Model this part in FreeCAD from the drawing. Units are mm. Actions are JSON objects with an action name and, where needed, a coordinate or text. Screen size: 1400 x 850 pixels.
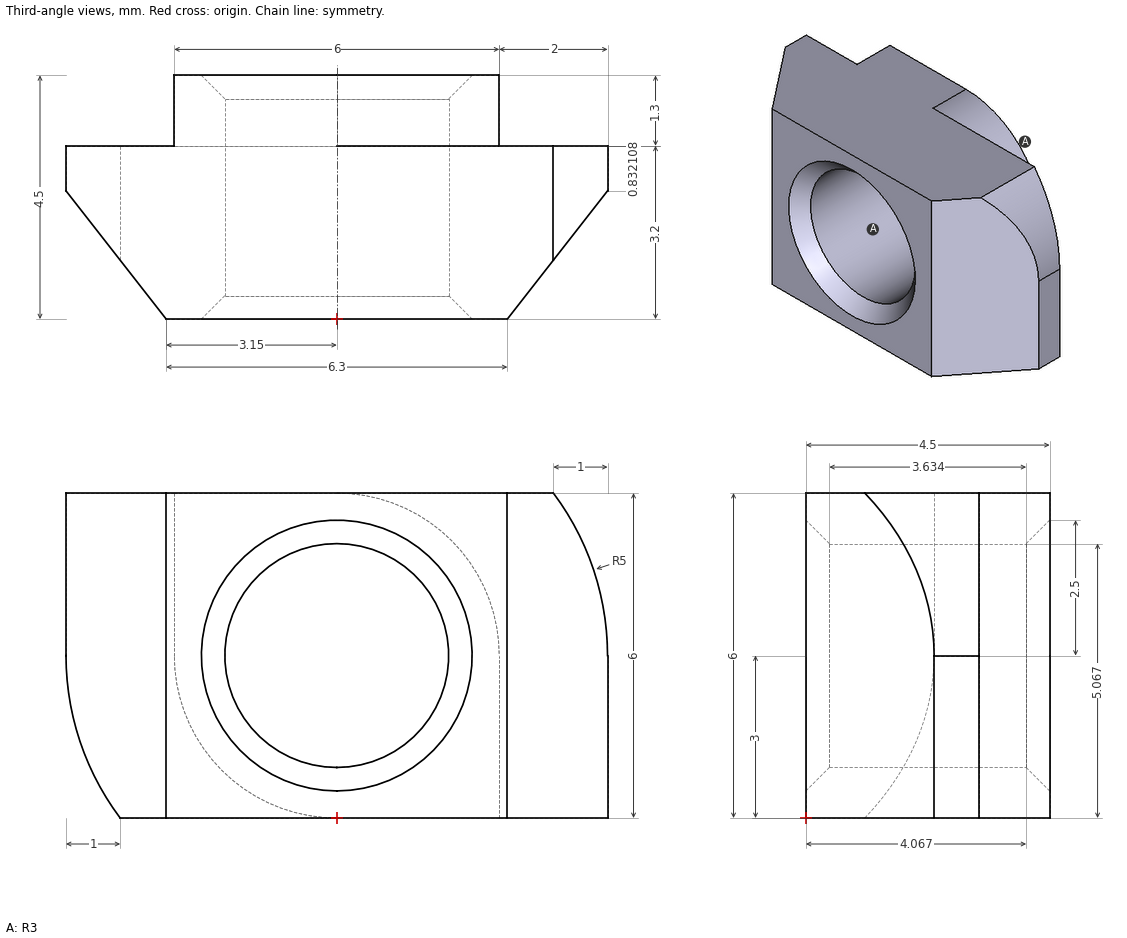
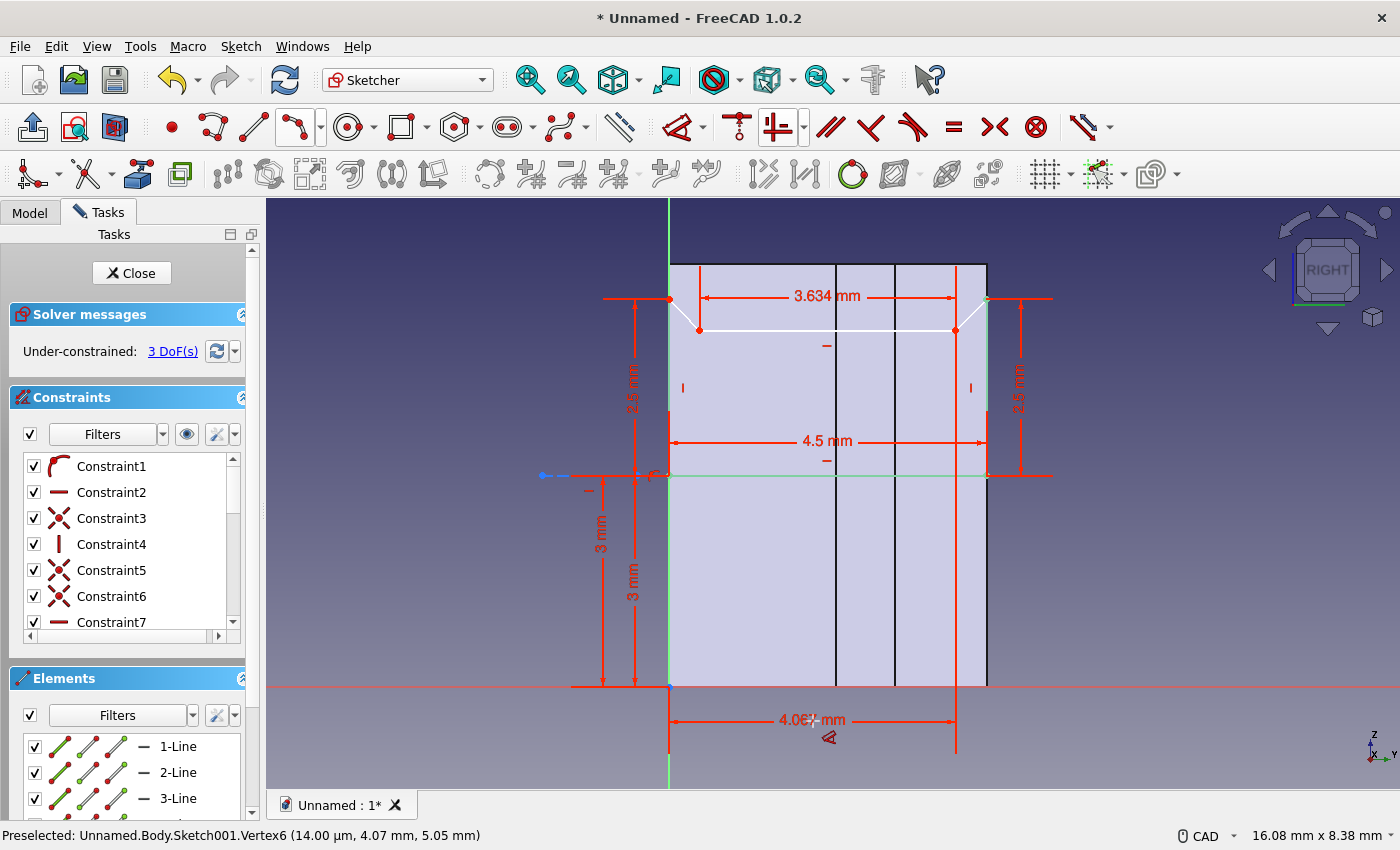
{"action": "left_click", "coordinate": [956, 331]}
{"action": "left_click", "coordinate": [990, 509]}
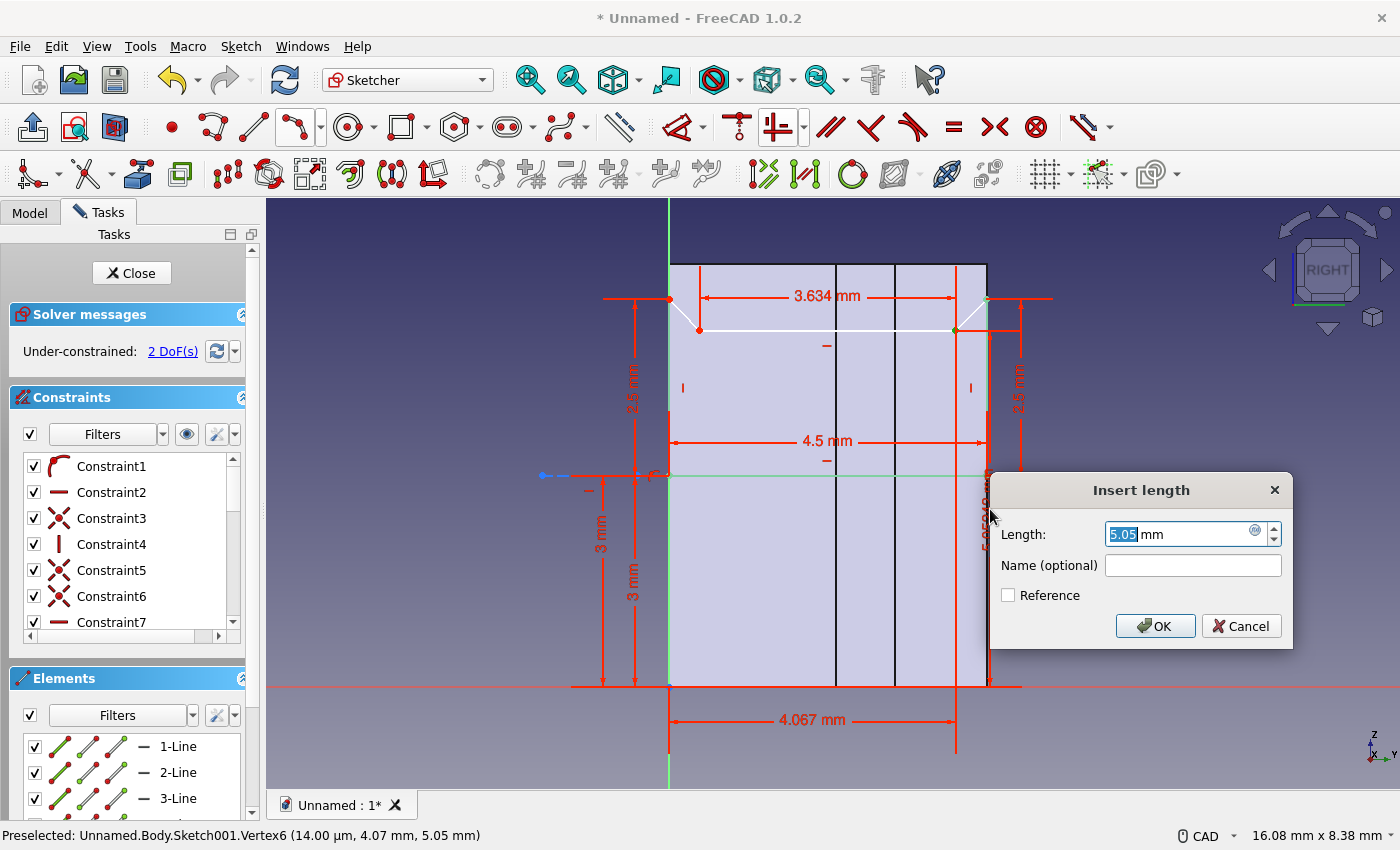
{"action": "type", "text": "5.067"}
{"action": "key", "text": "Return"}
{"action": "key", "text": "Escape"}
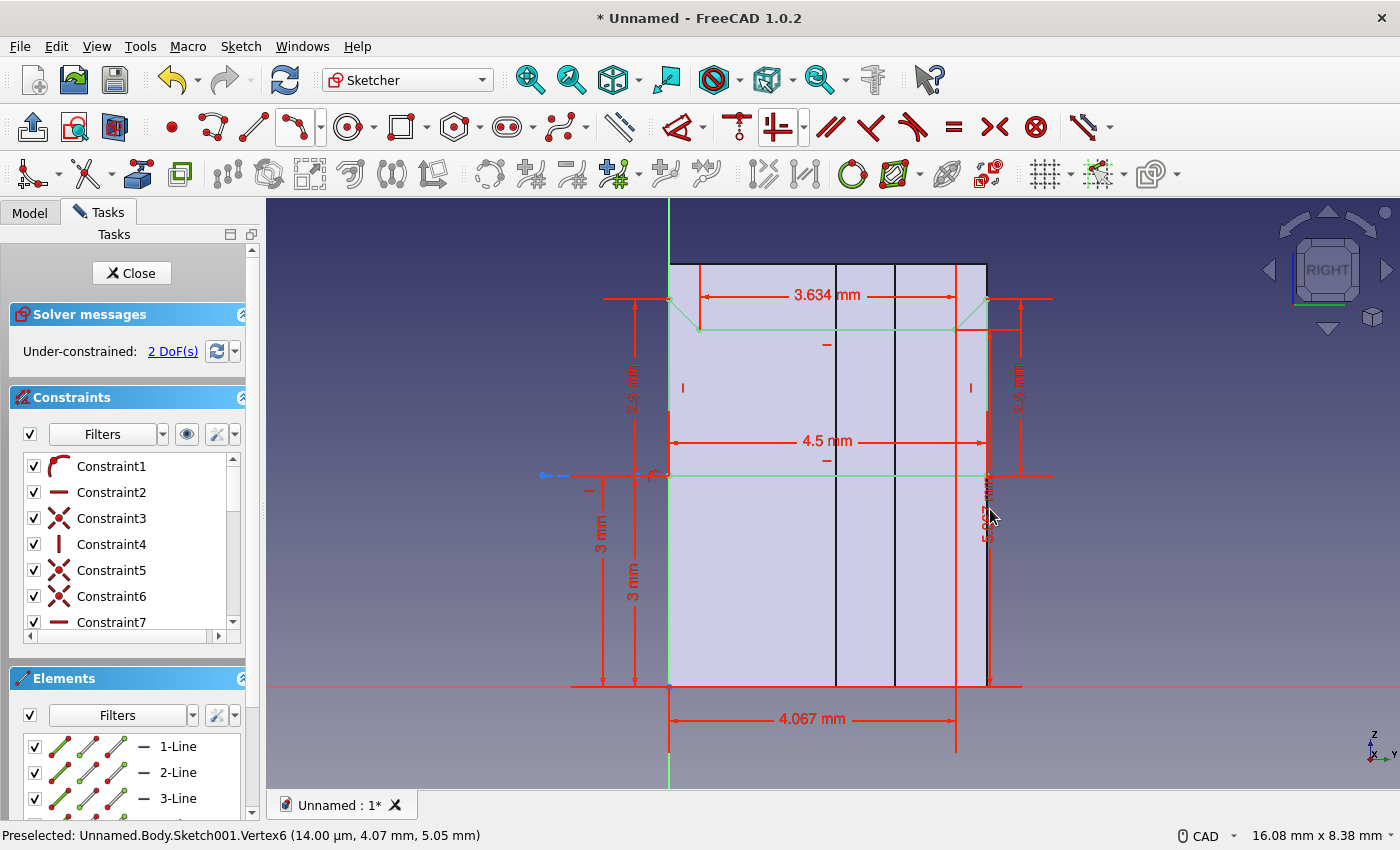
{"action": "left_click", "coordinate": [132, 273]}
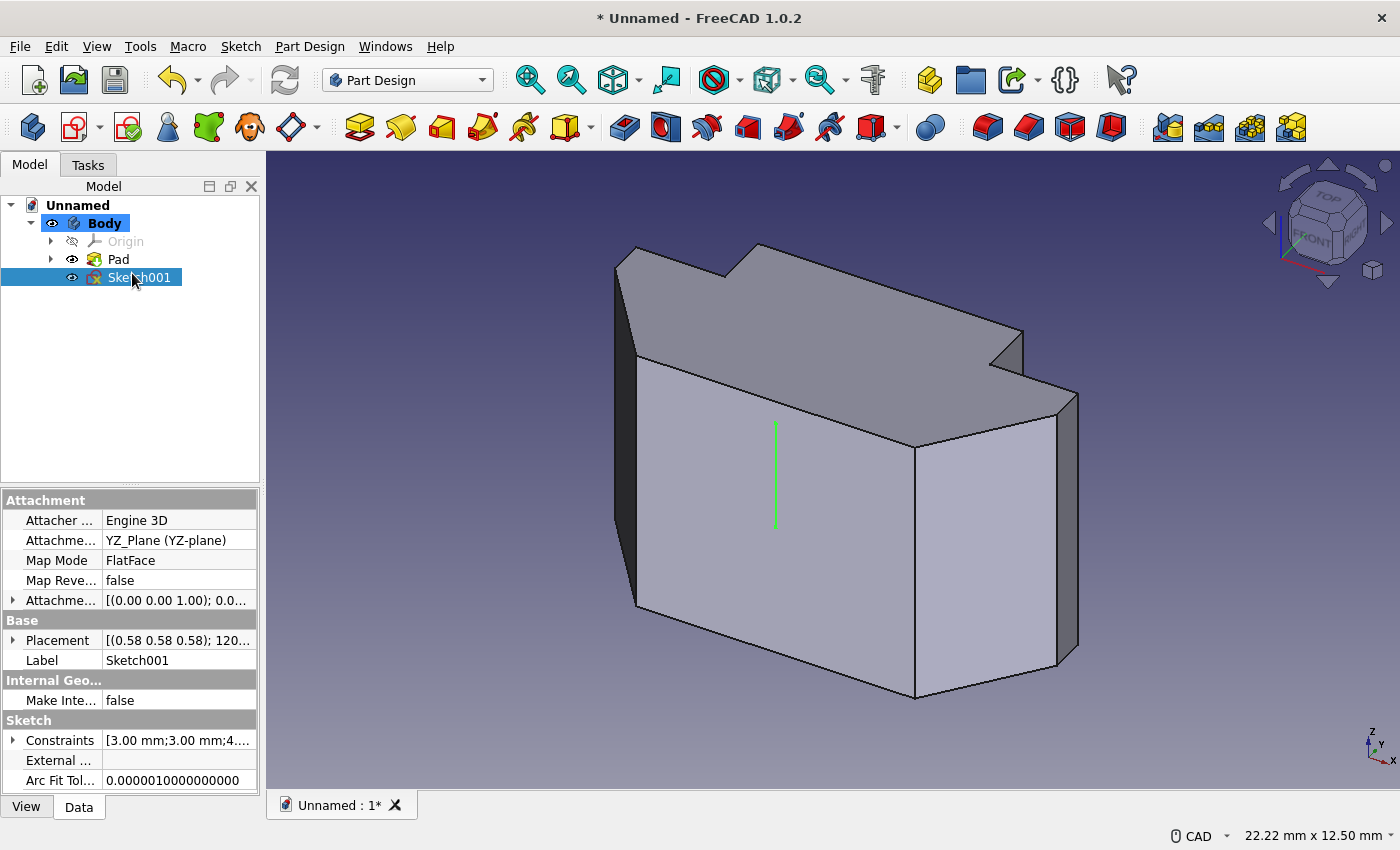
{"action": "left_click", "coordinate": [707, 128]}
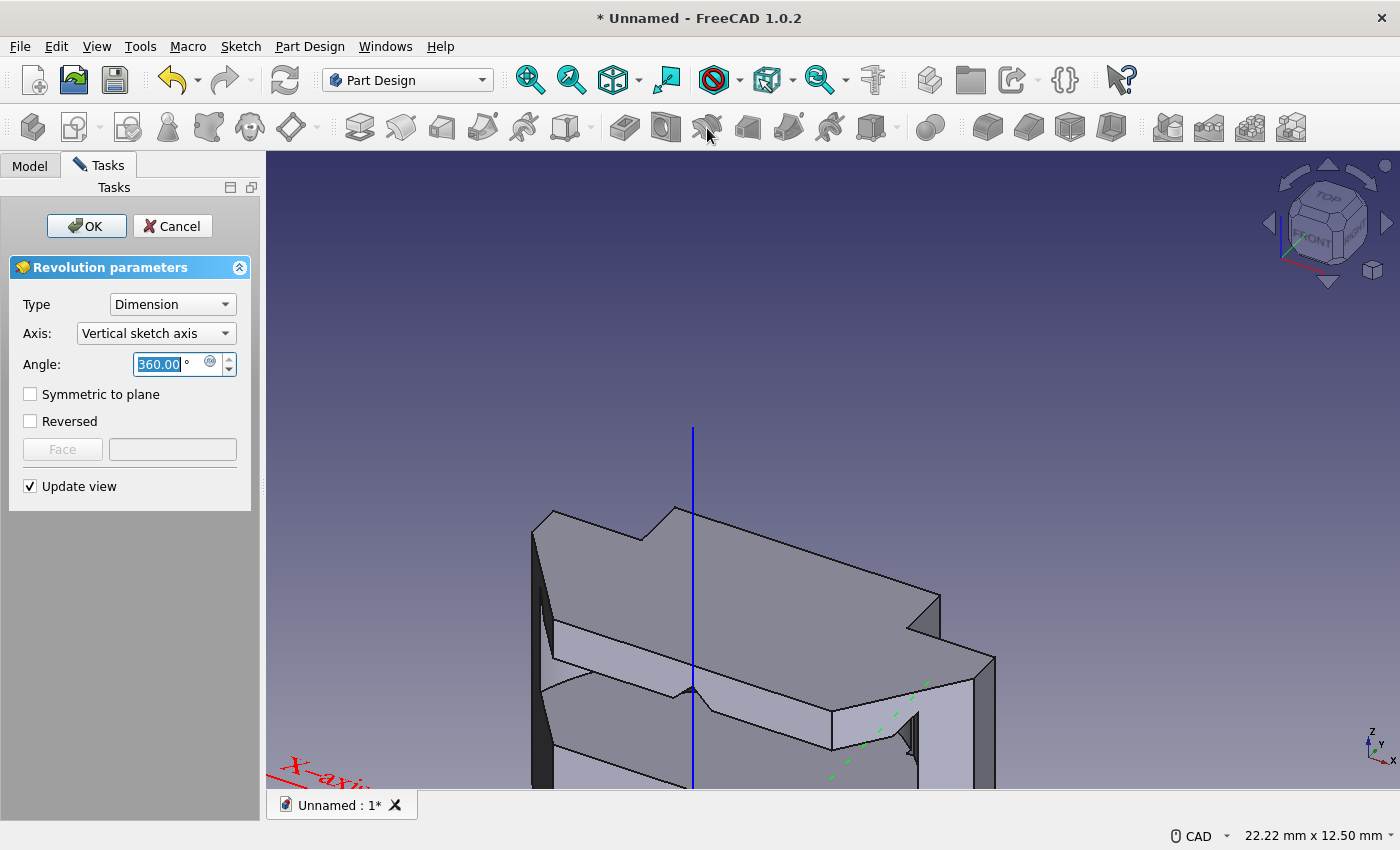
{"action": "left_click", "coordinate": [157, 334]}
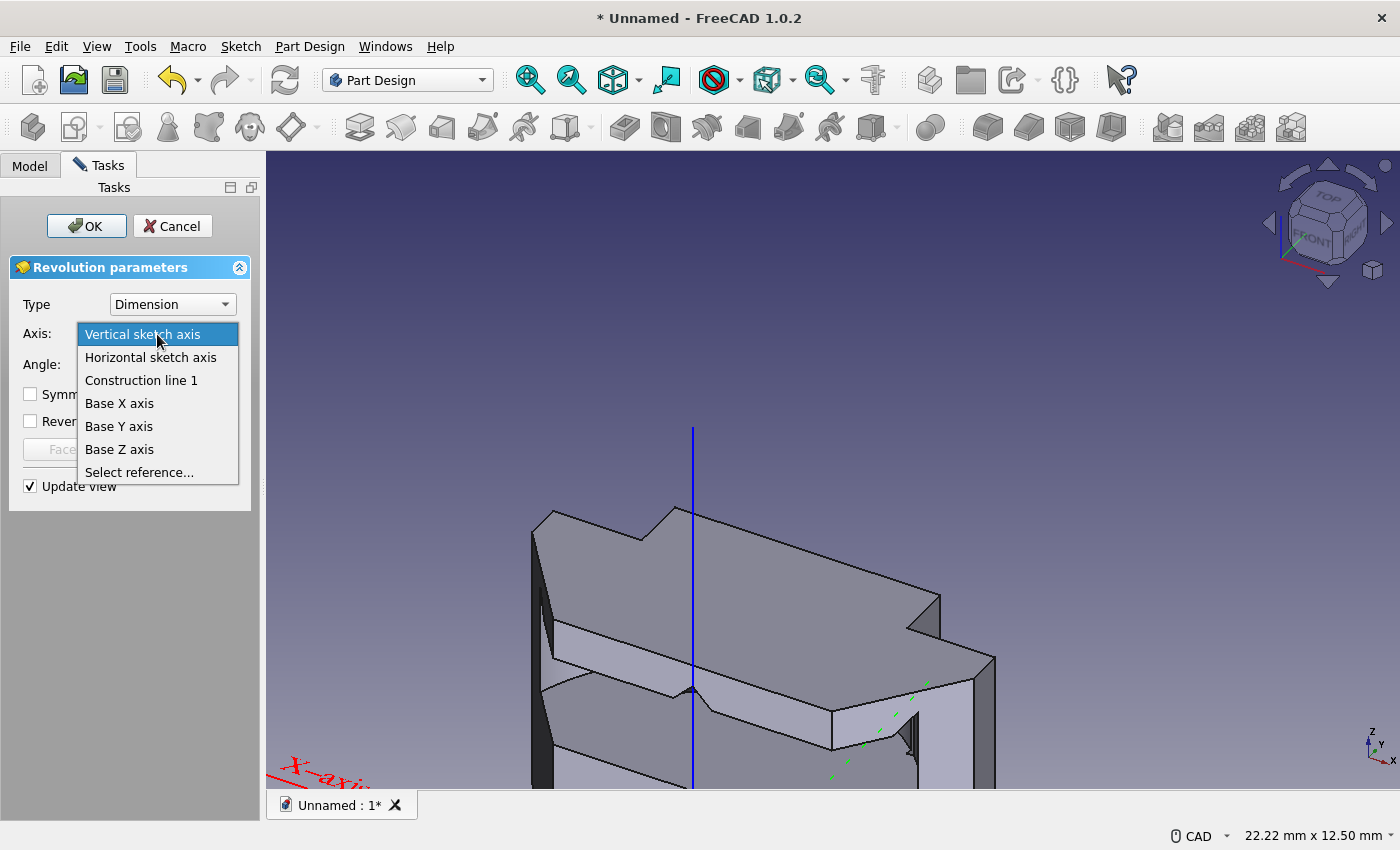
{"action": "left_click", "coordinate": [156, 380]}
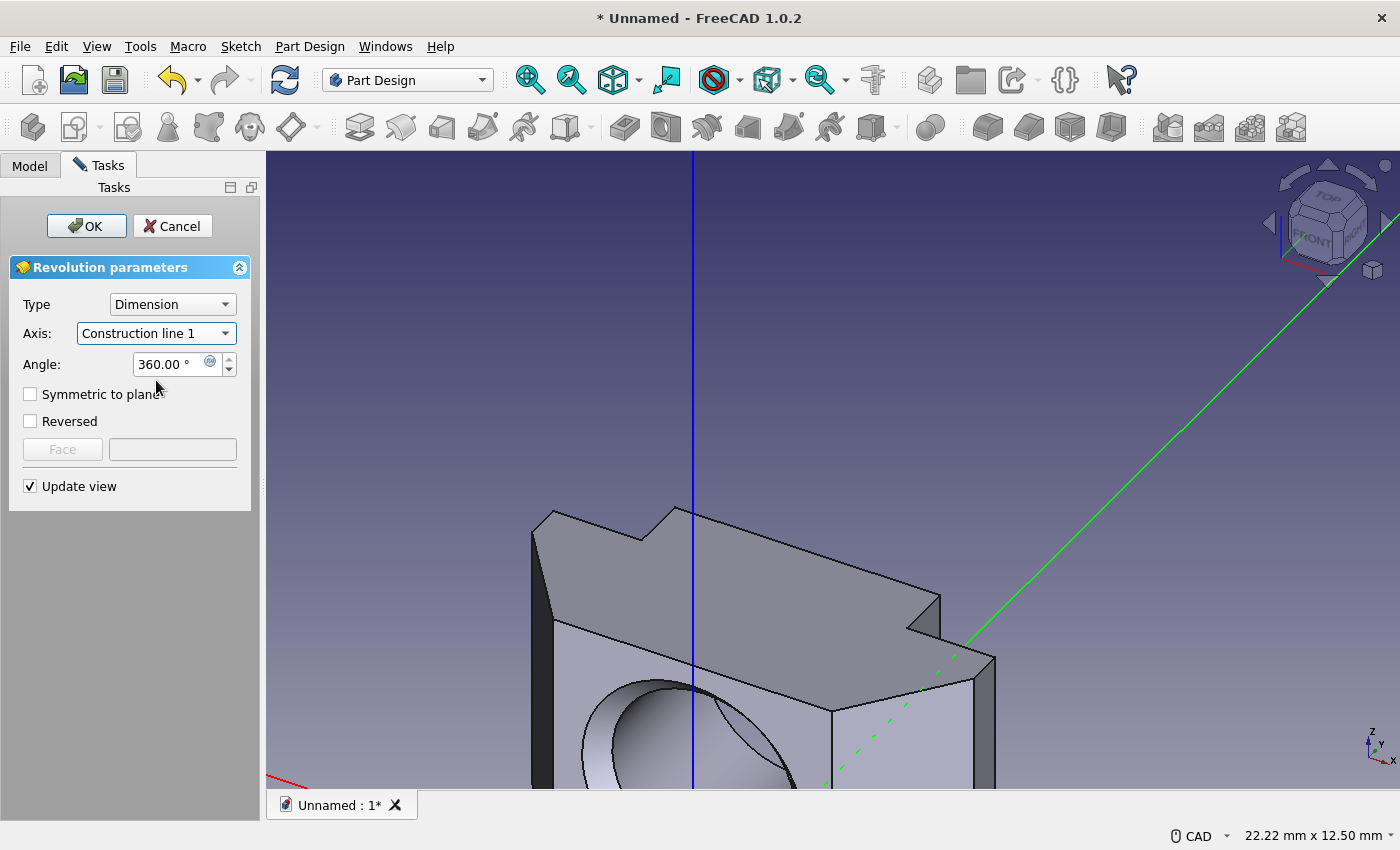
{"action": "left_click", "coordinate": [87, 226]}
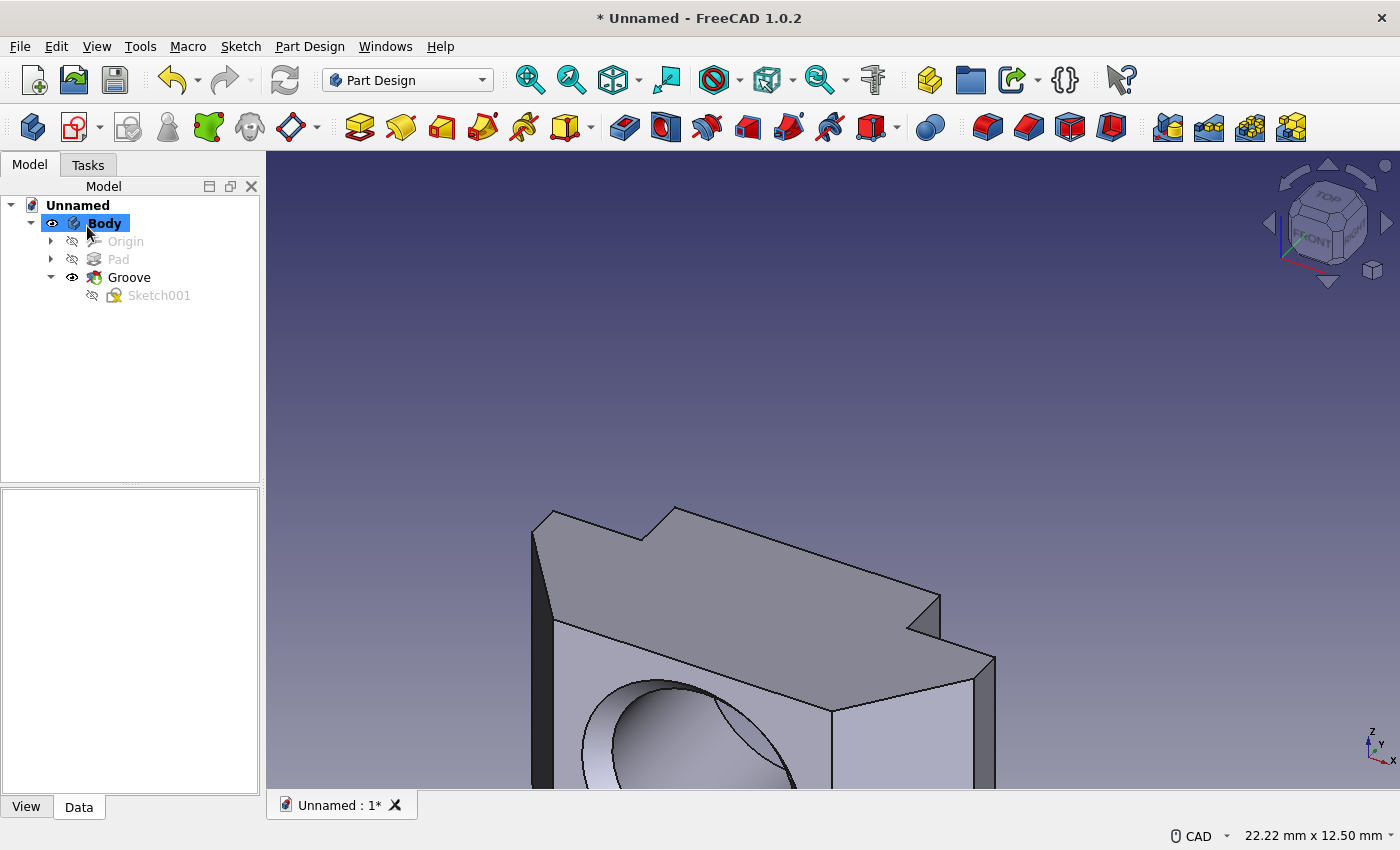
{"action": "left_click", "coordinate": [531, 80]}